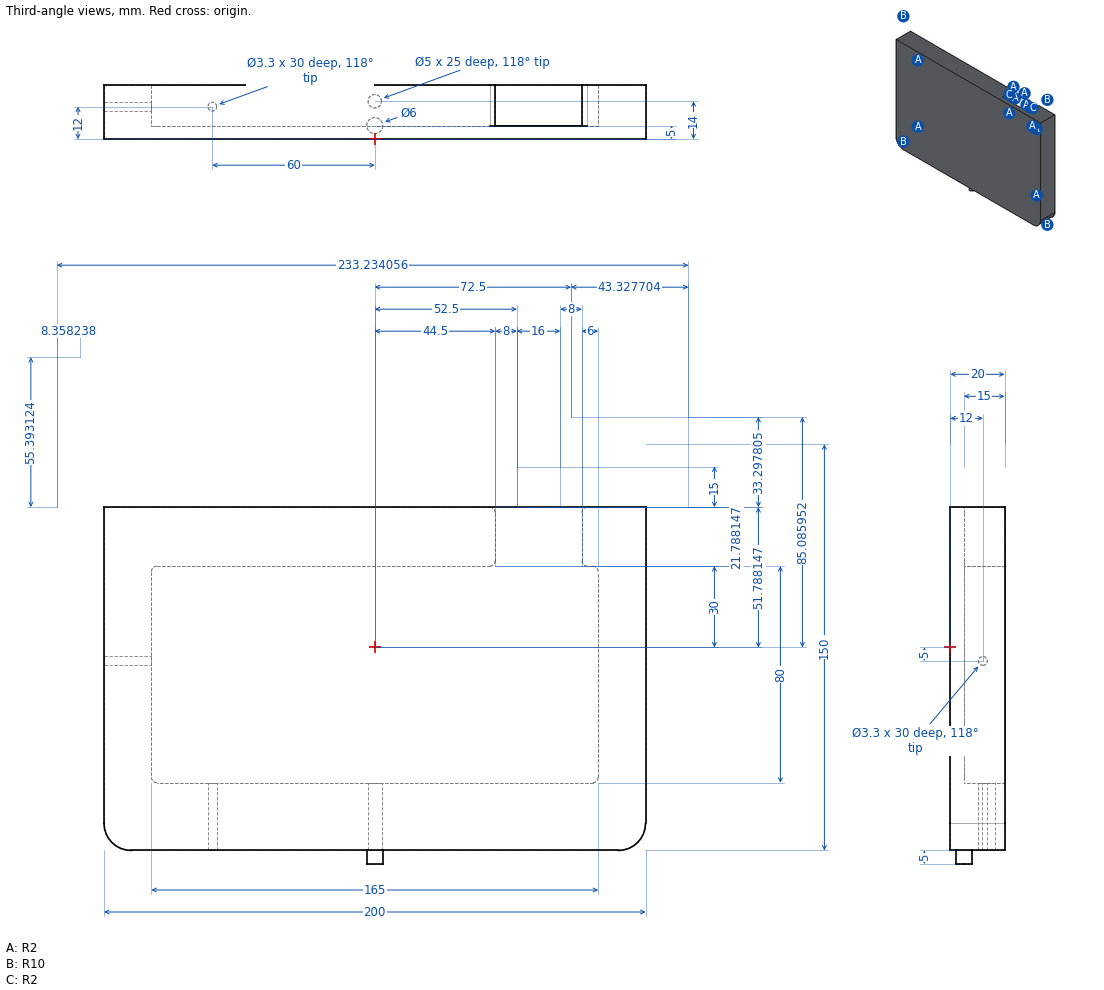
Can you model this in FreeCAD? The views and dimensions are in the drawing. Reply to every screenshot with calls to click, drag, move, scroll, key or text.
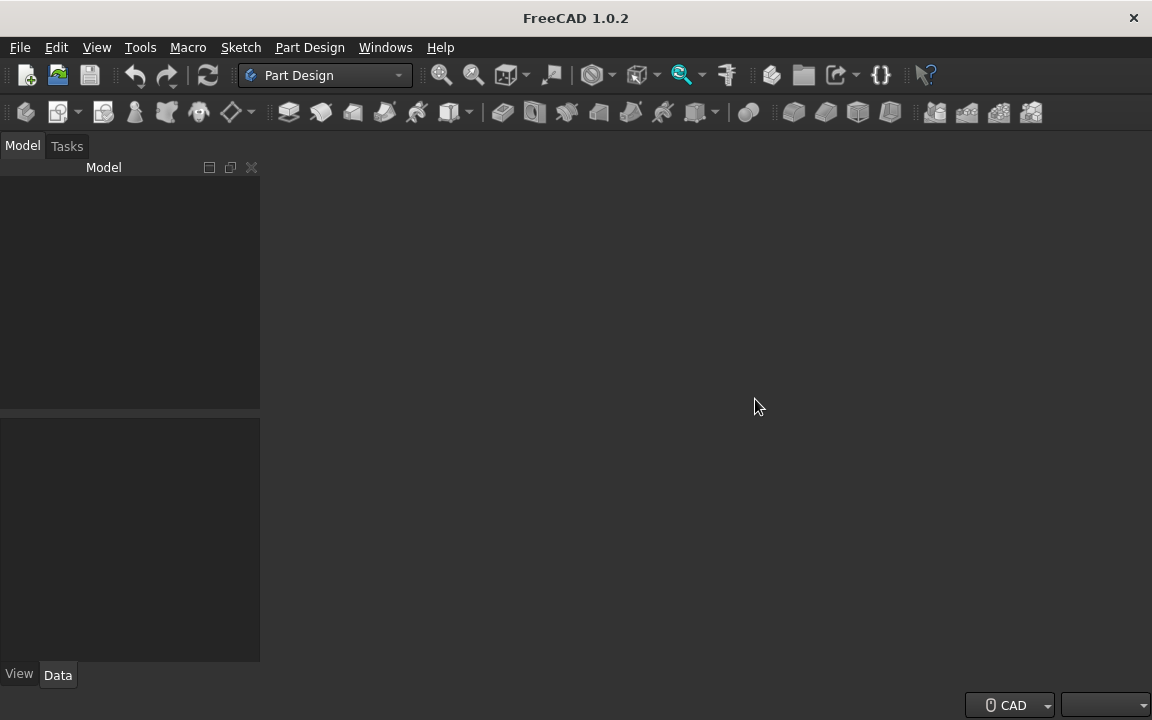
key(ctrl+n)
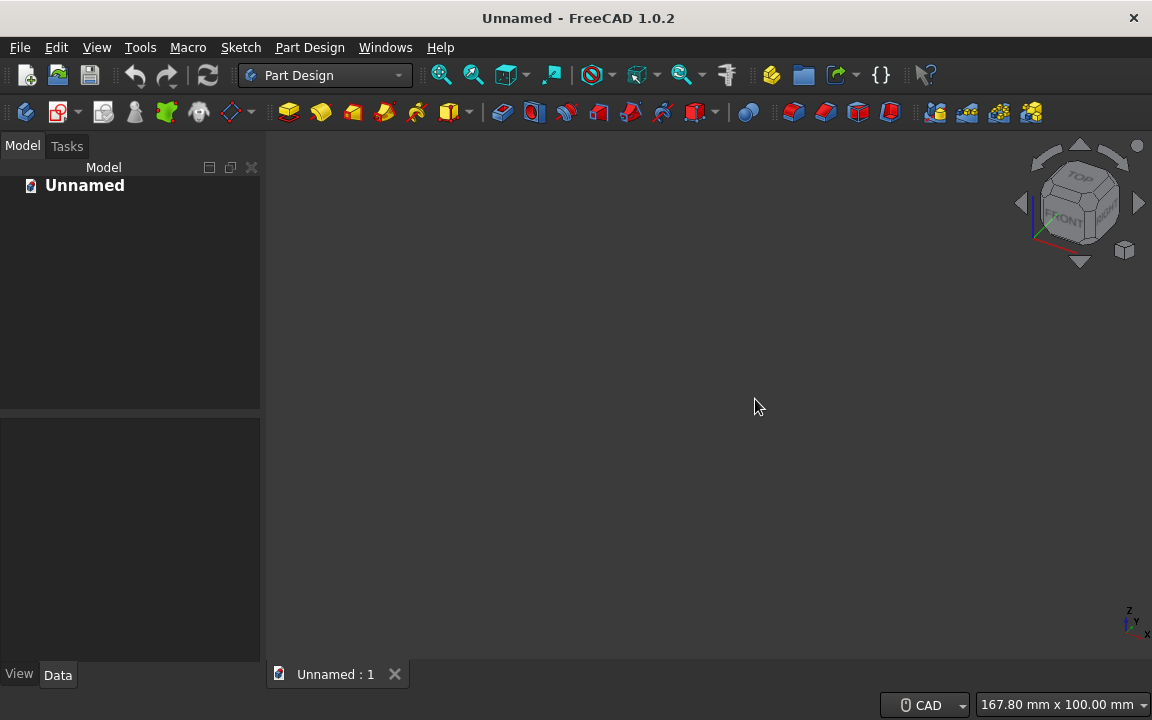
click(58, 112)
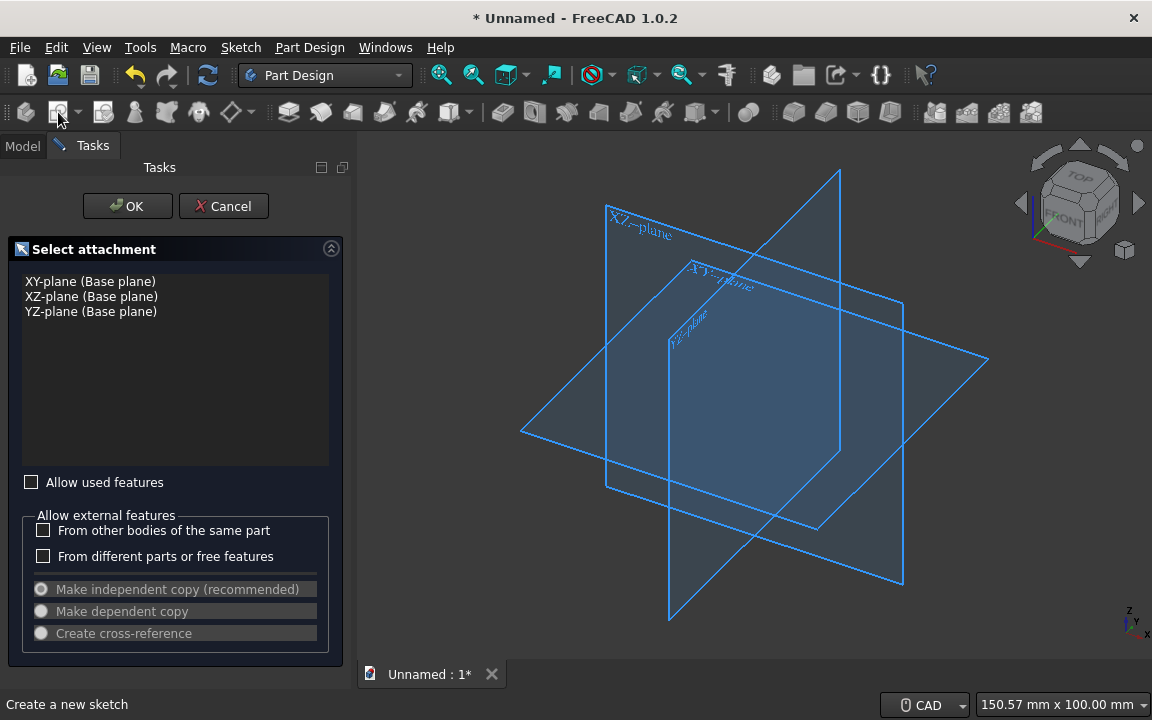
click(82, 296)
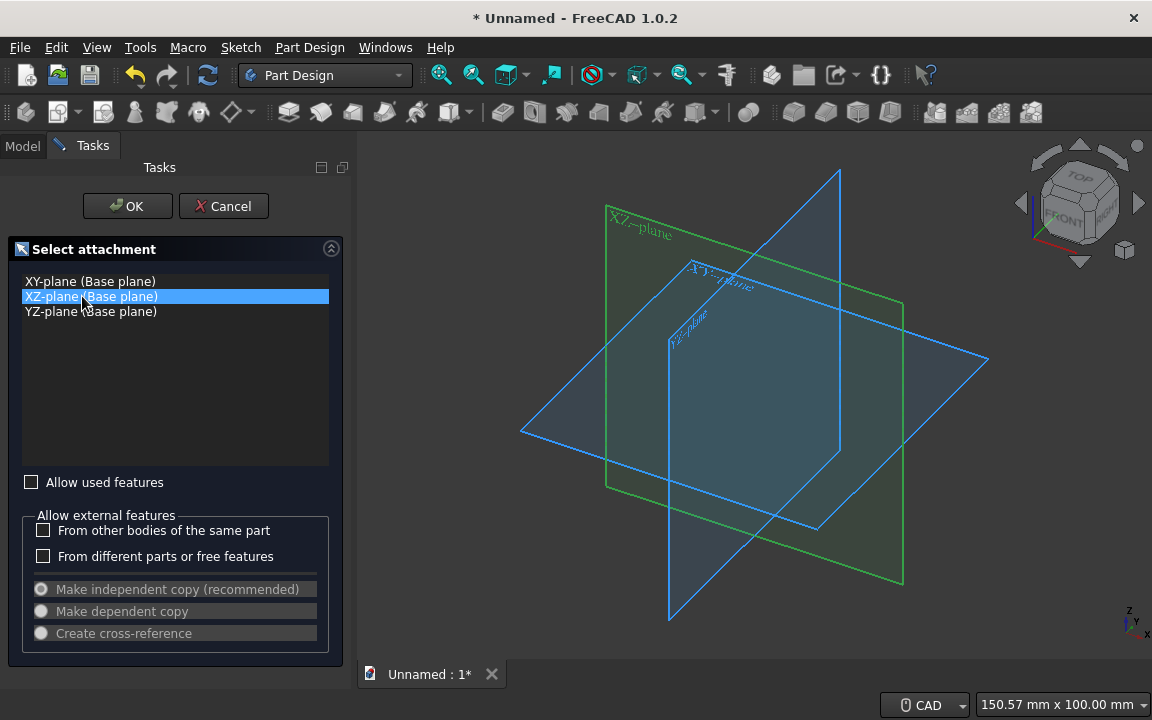
click(128, 206)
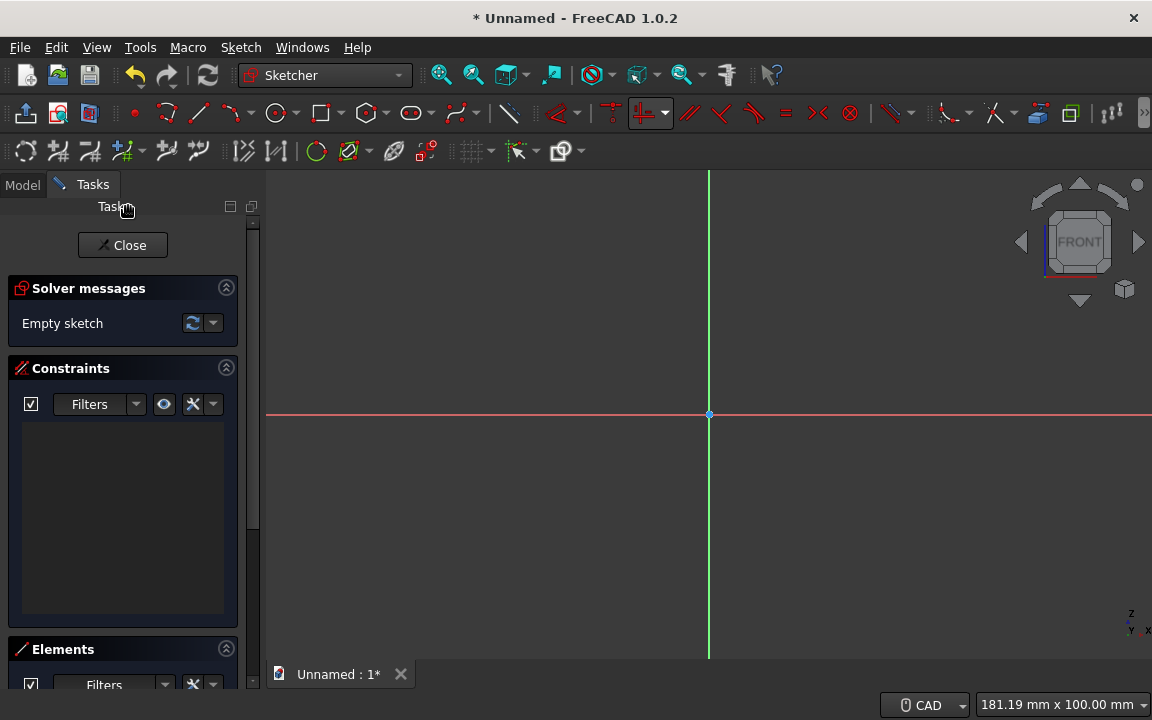
scroll(585, 414, down, 4)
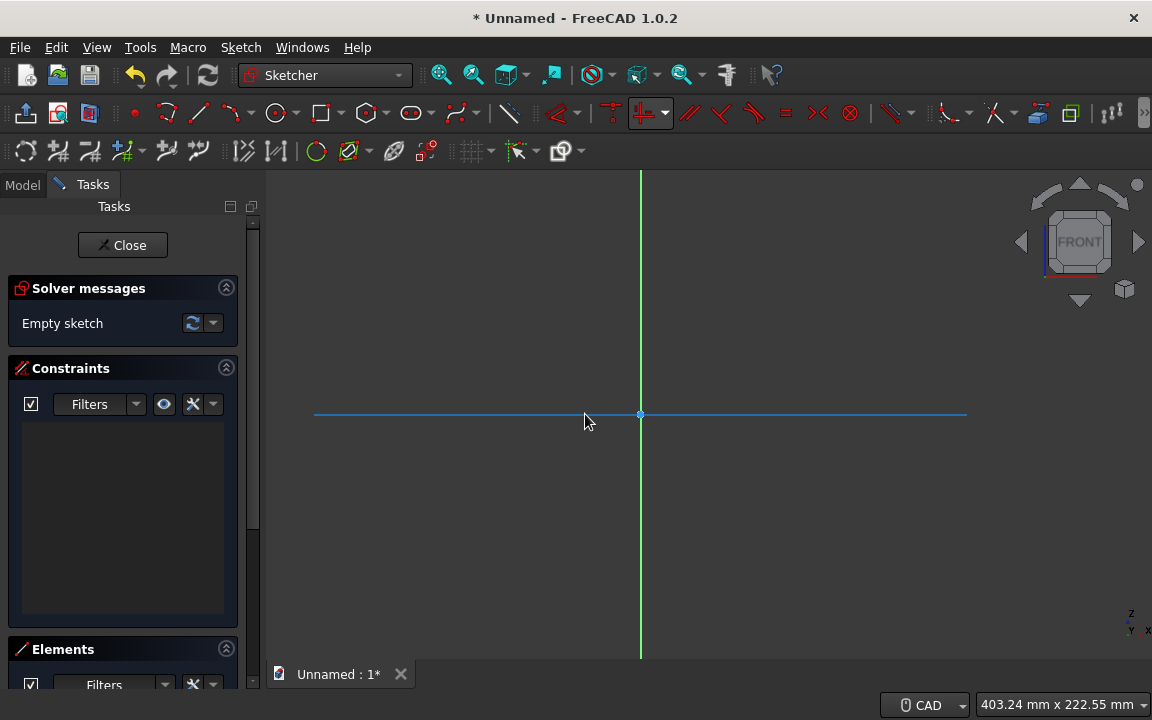
click(344, 114)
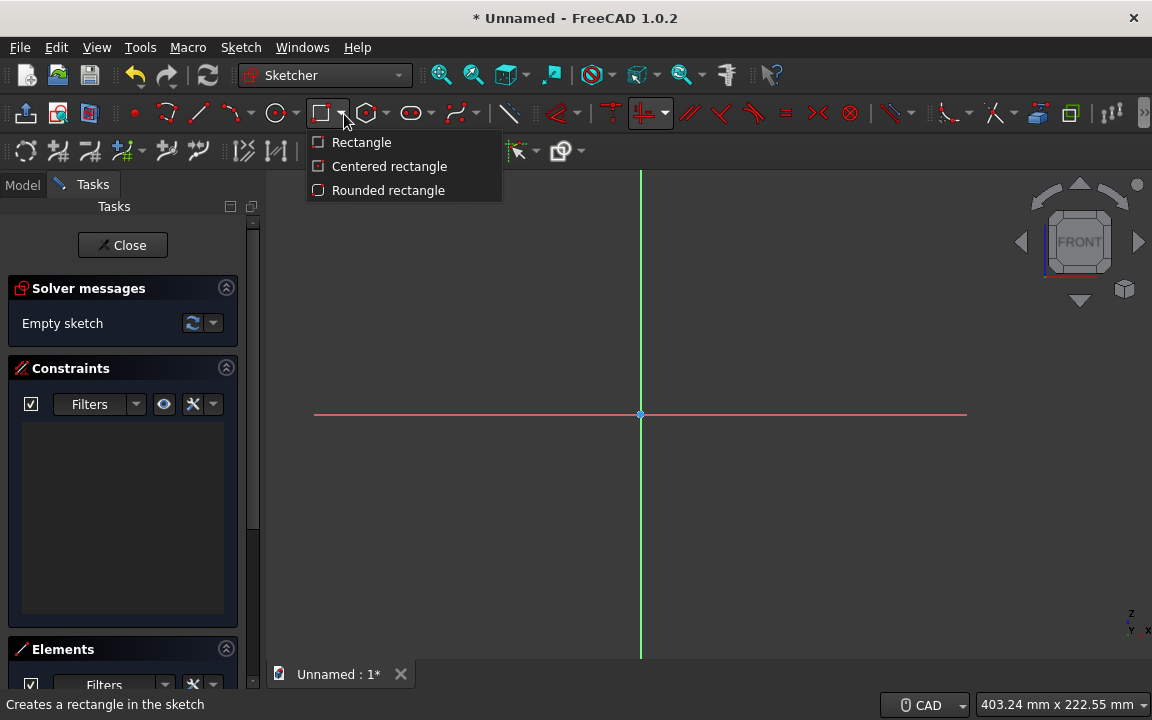
click(404, 166)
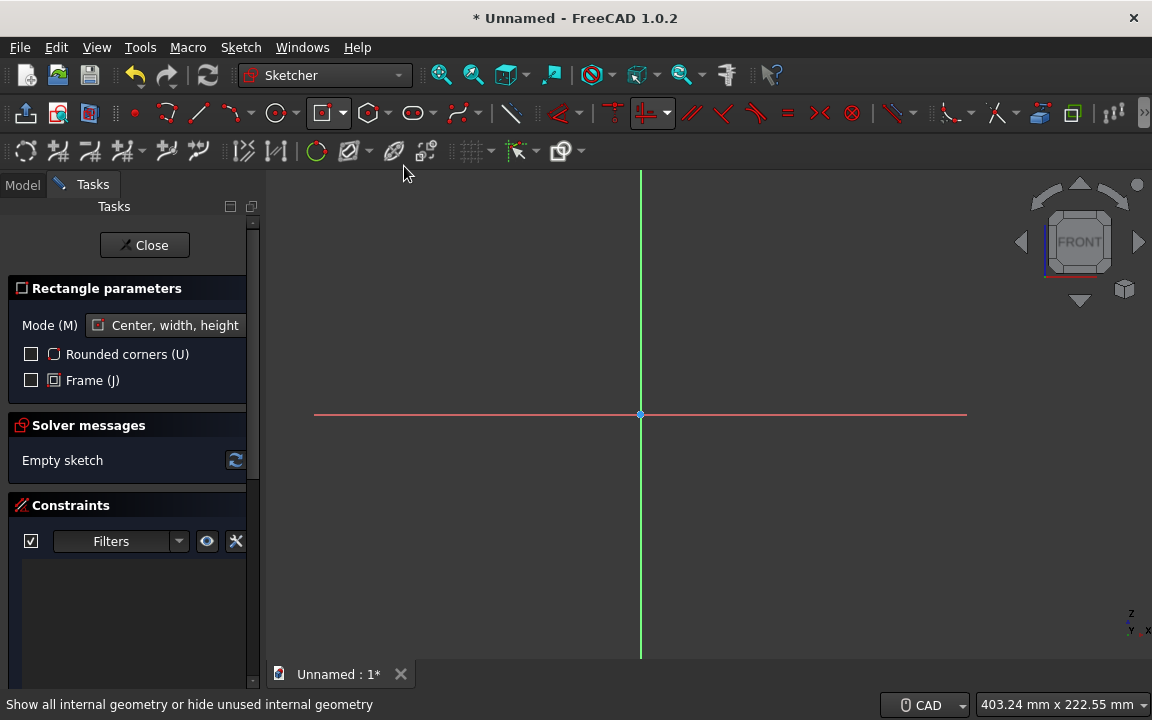
click(641, 414)
click(861, 250)
key(Escape)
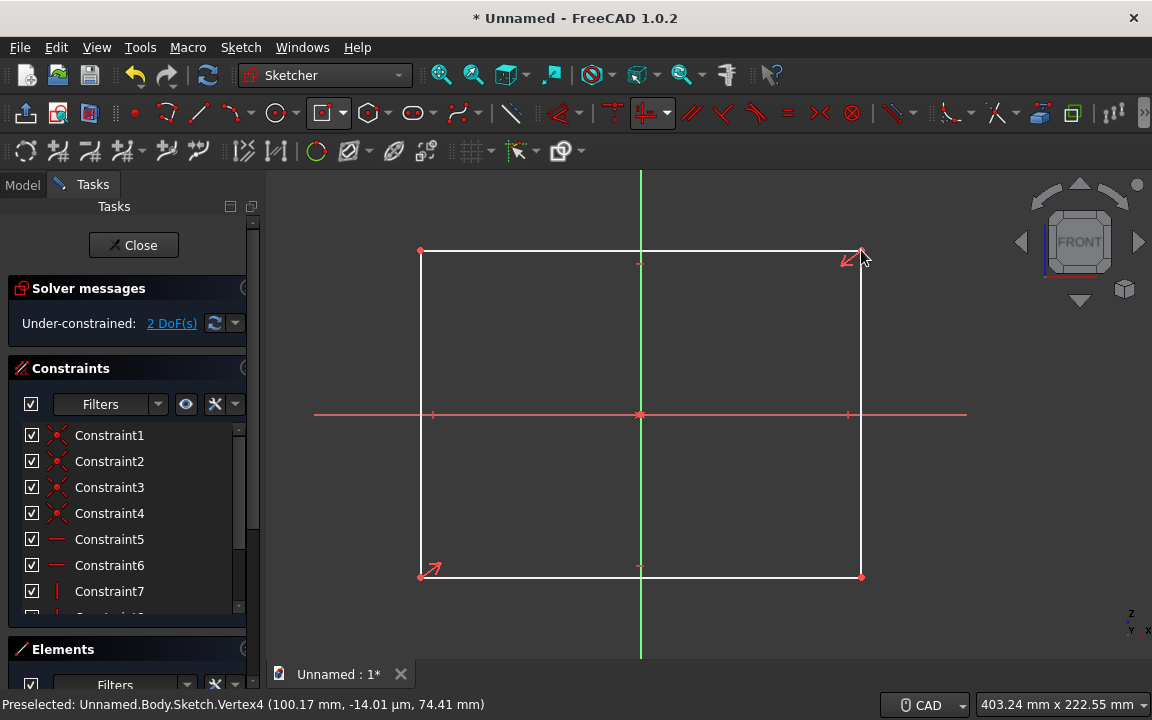
key(d)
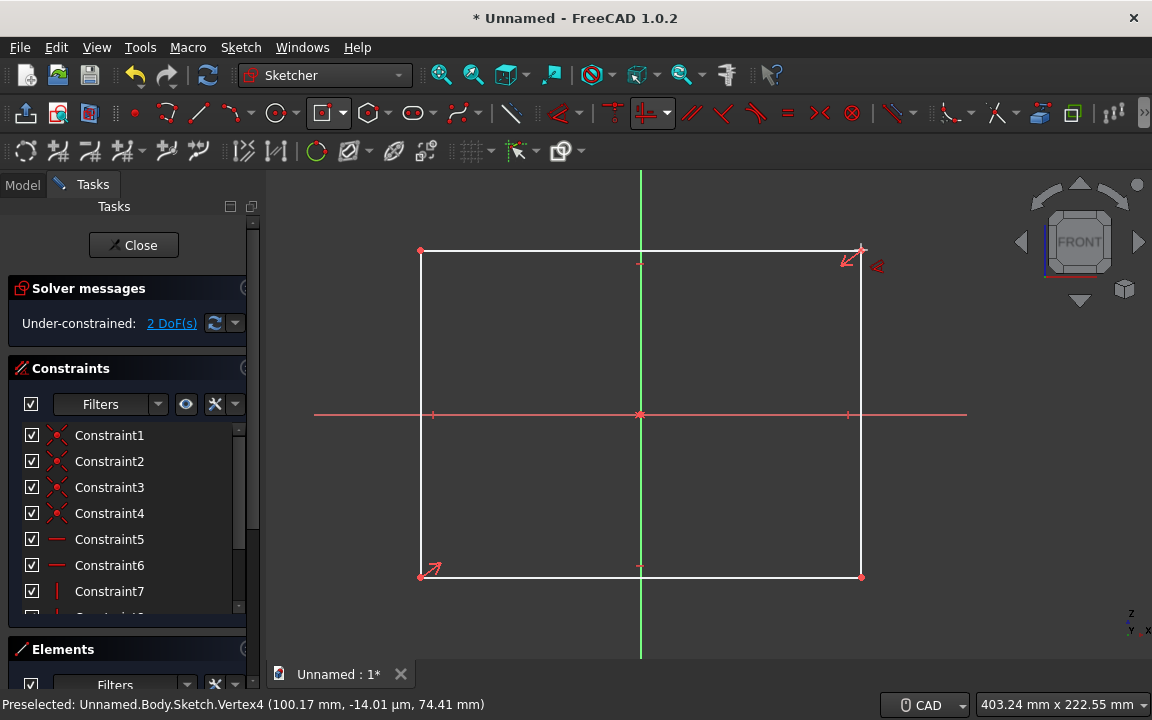
click(553, 578)
click(540, 612)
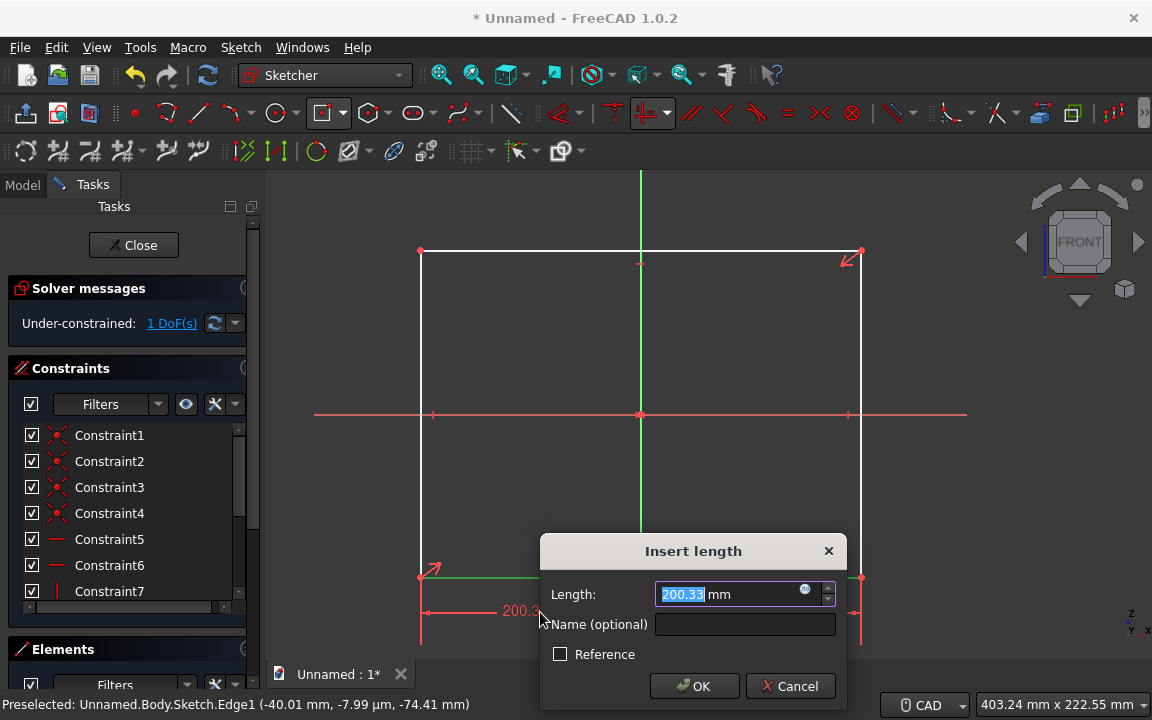
text(200)
key(Return)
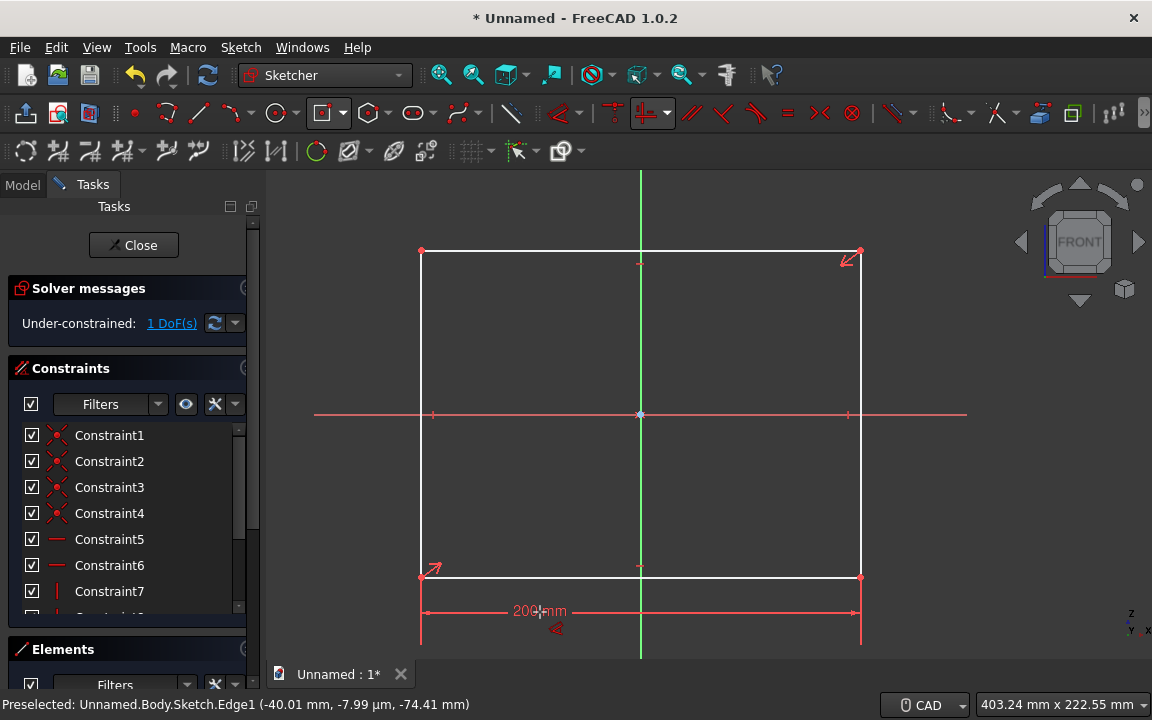
click(861, 480)
click(895, 339)